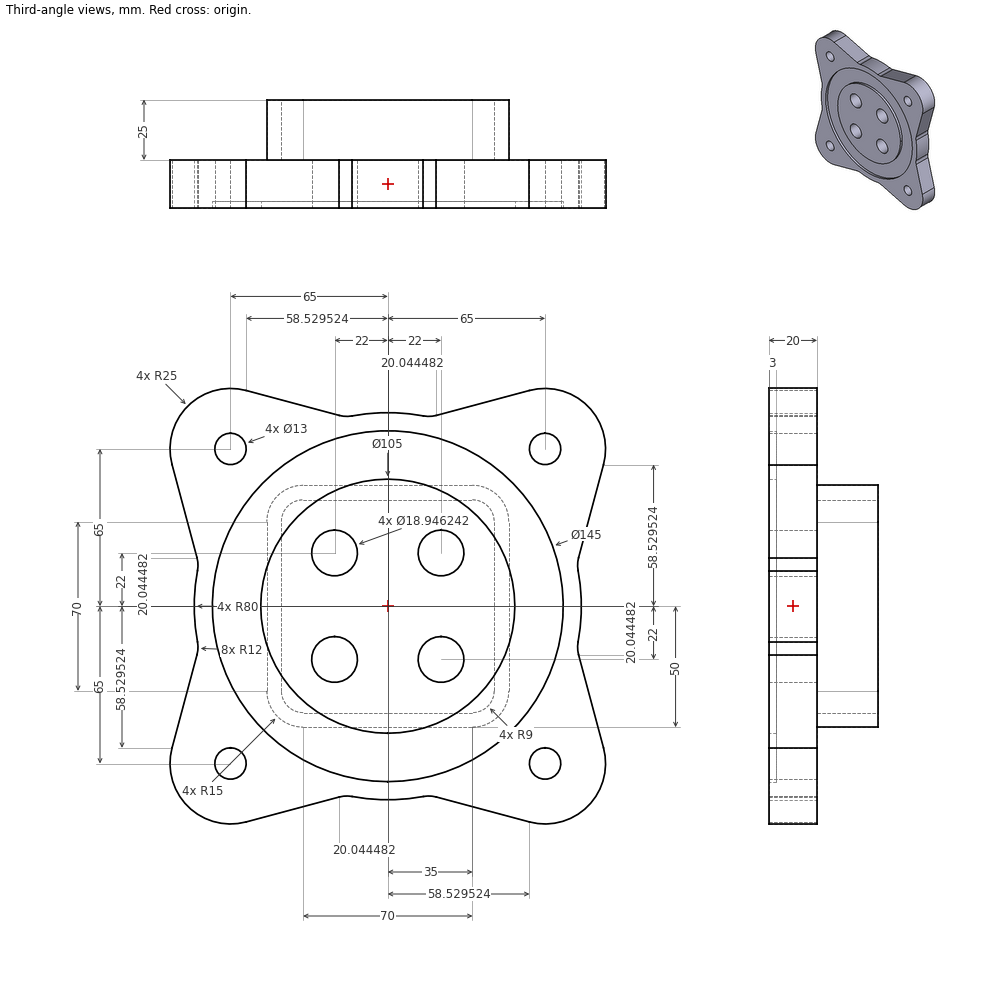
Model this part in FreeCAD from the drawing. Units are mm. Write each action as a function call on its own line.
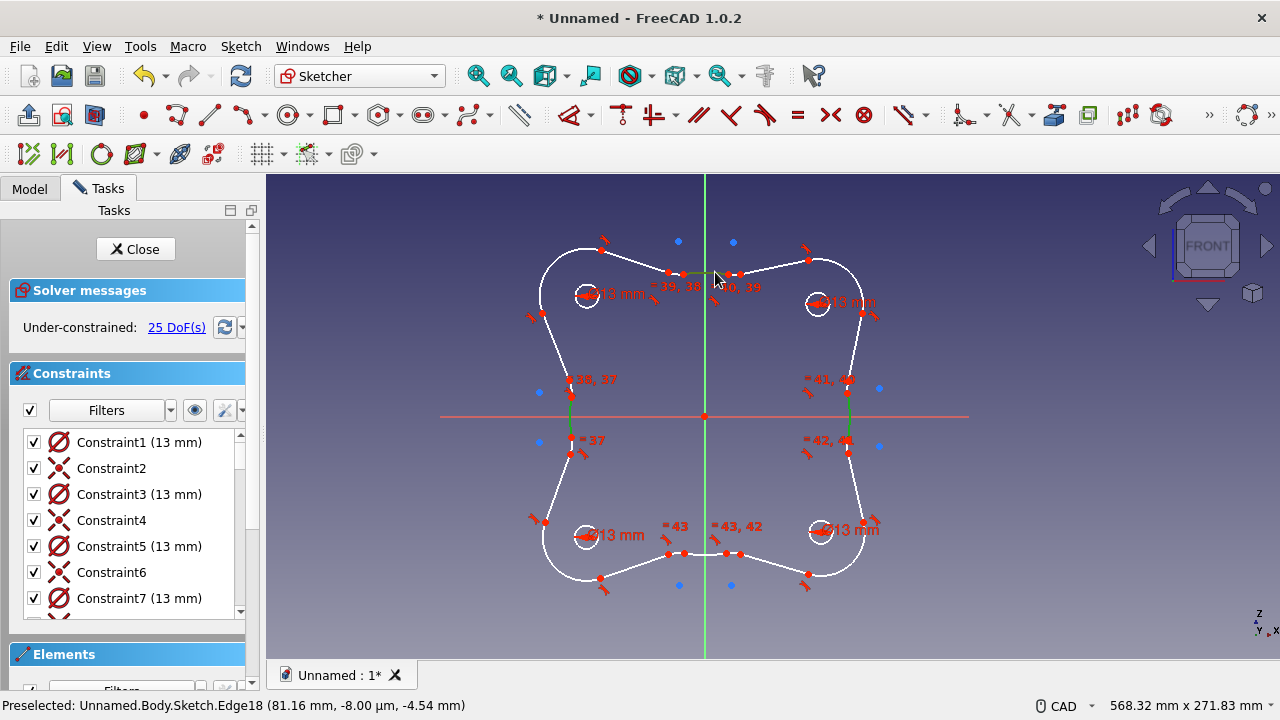
scroll(697, 555, up, 3)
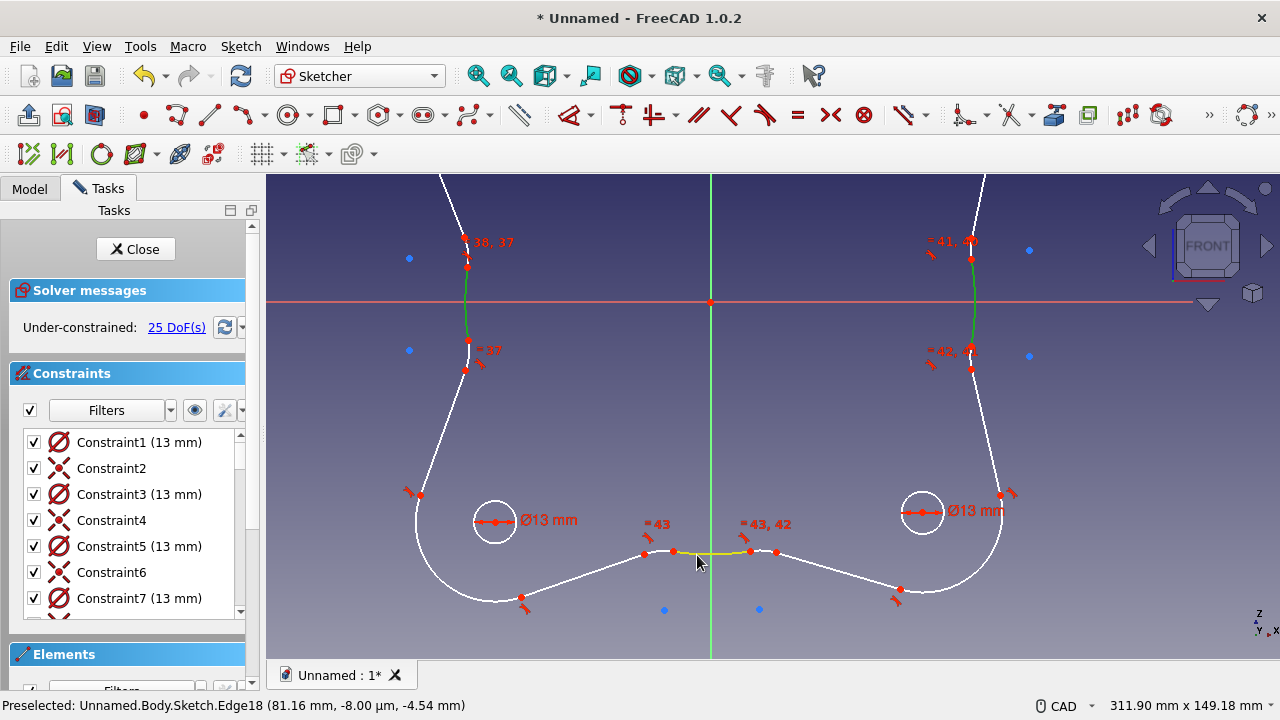
click(696, 554)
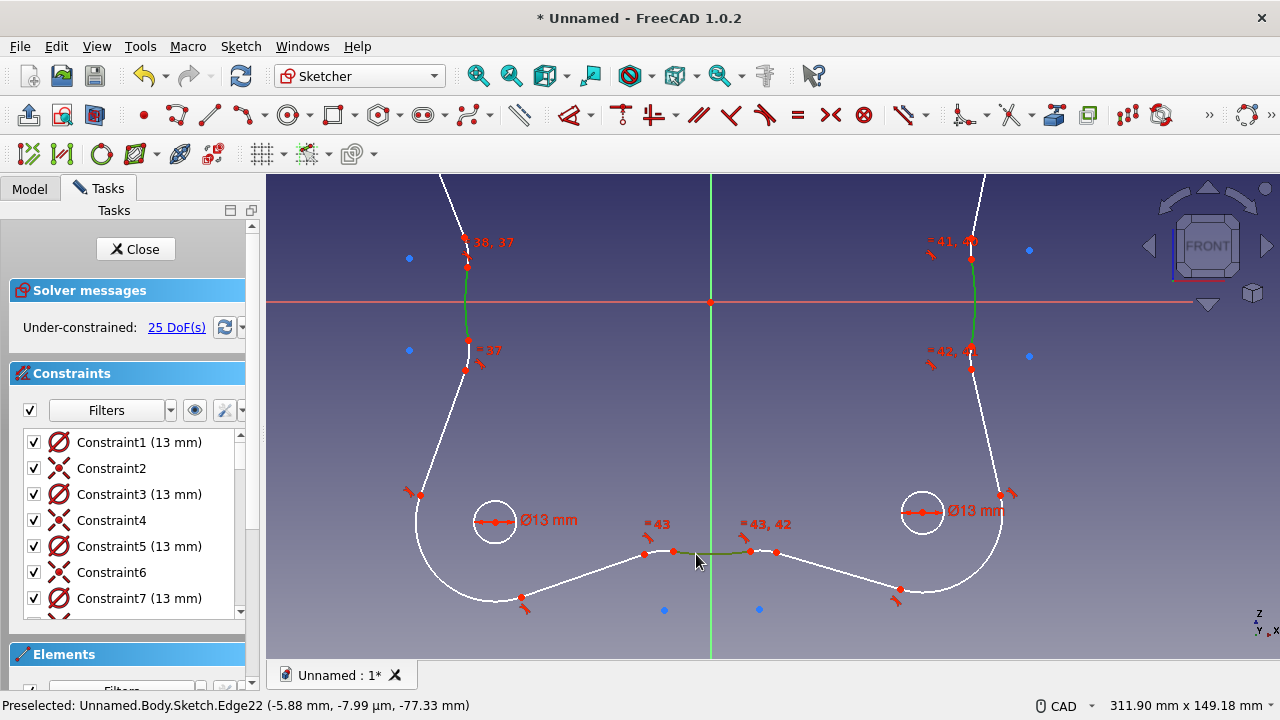
click(798, 116)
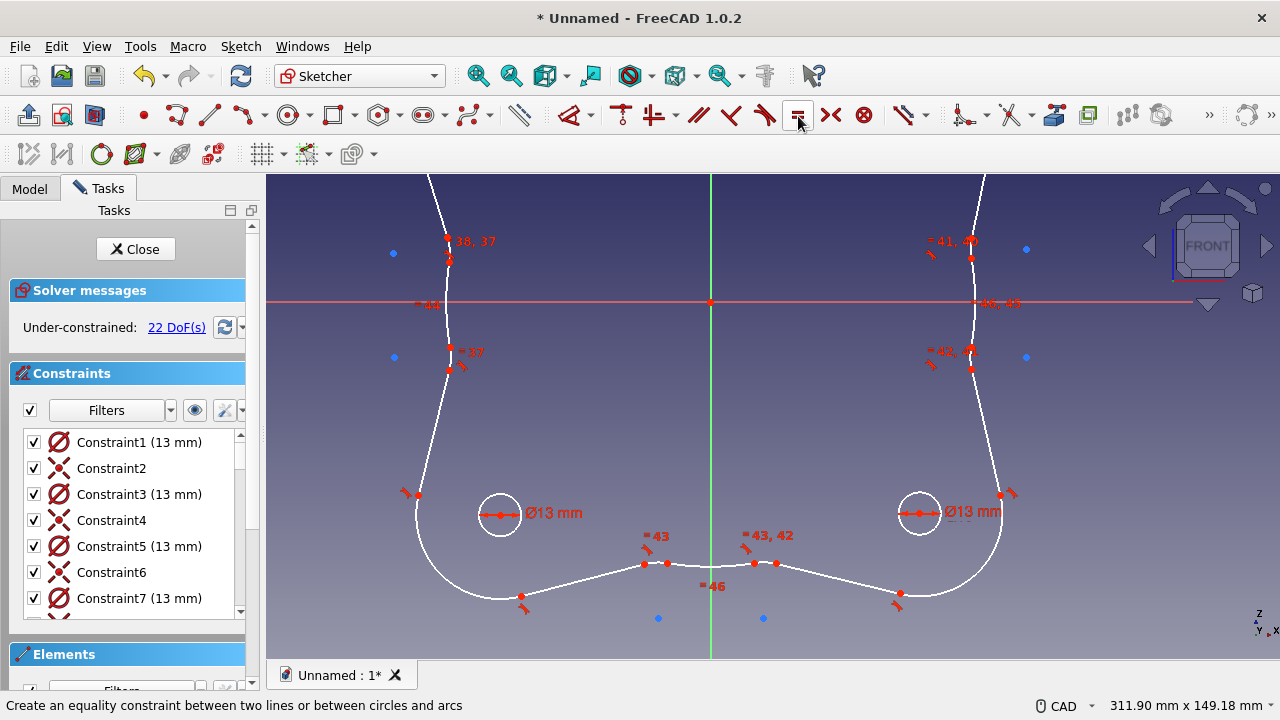
scroll(697, 555, down, 3)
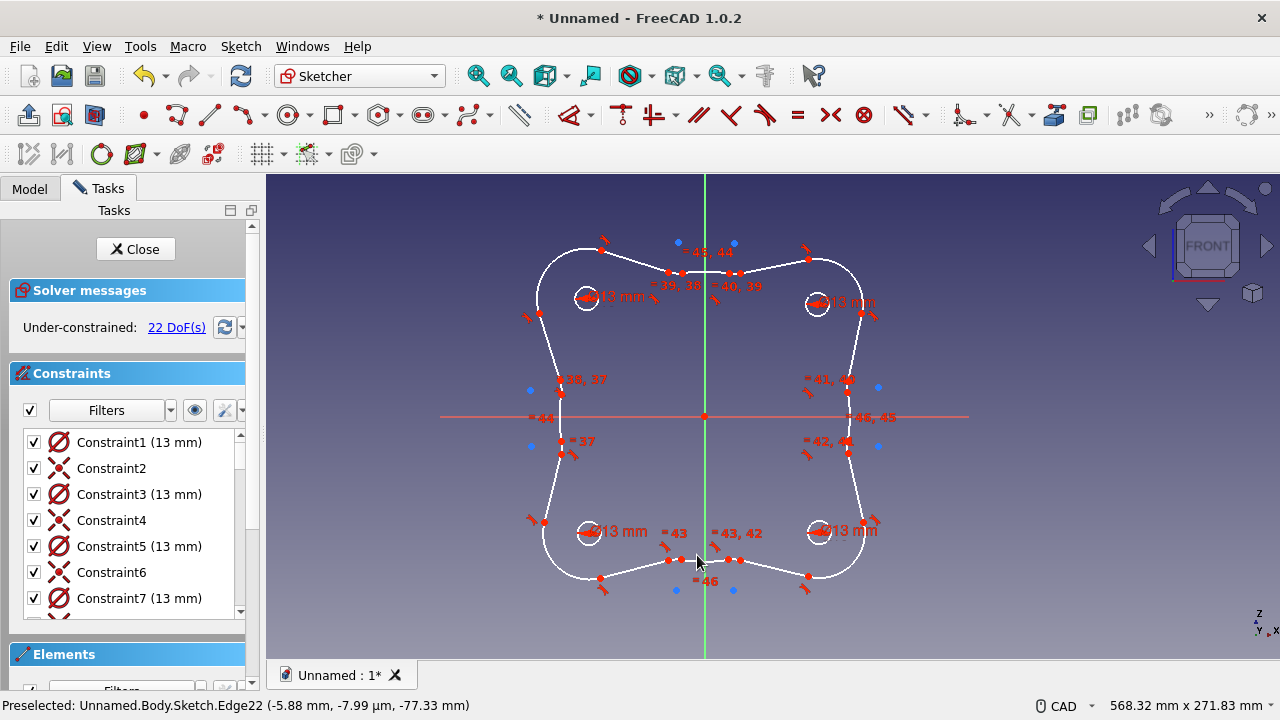
click(570, 252)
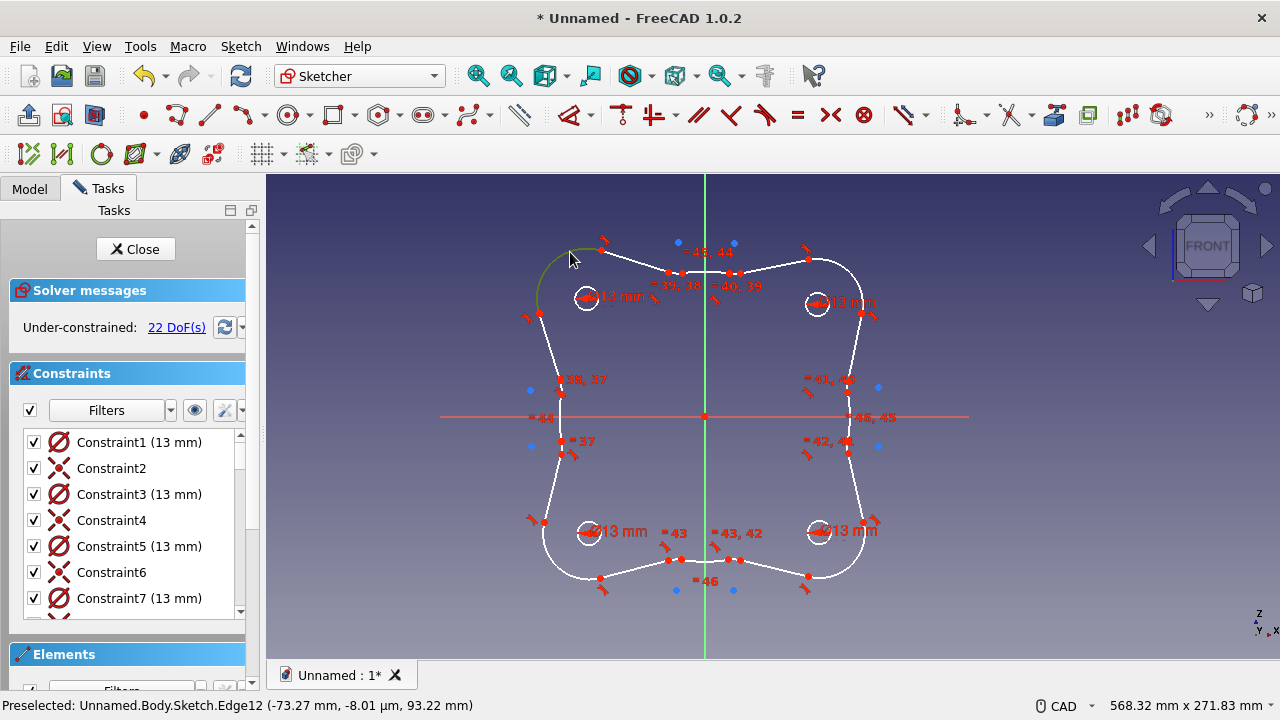
click(859, 287)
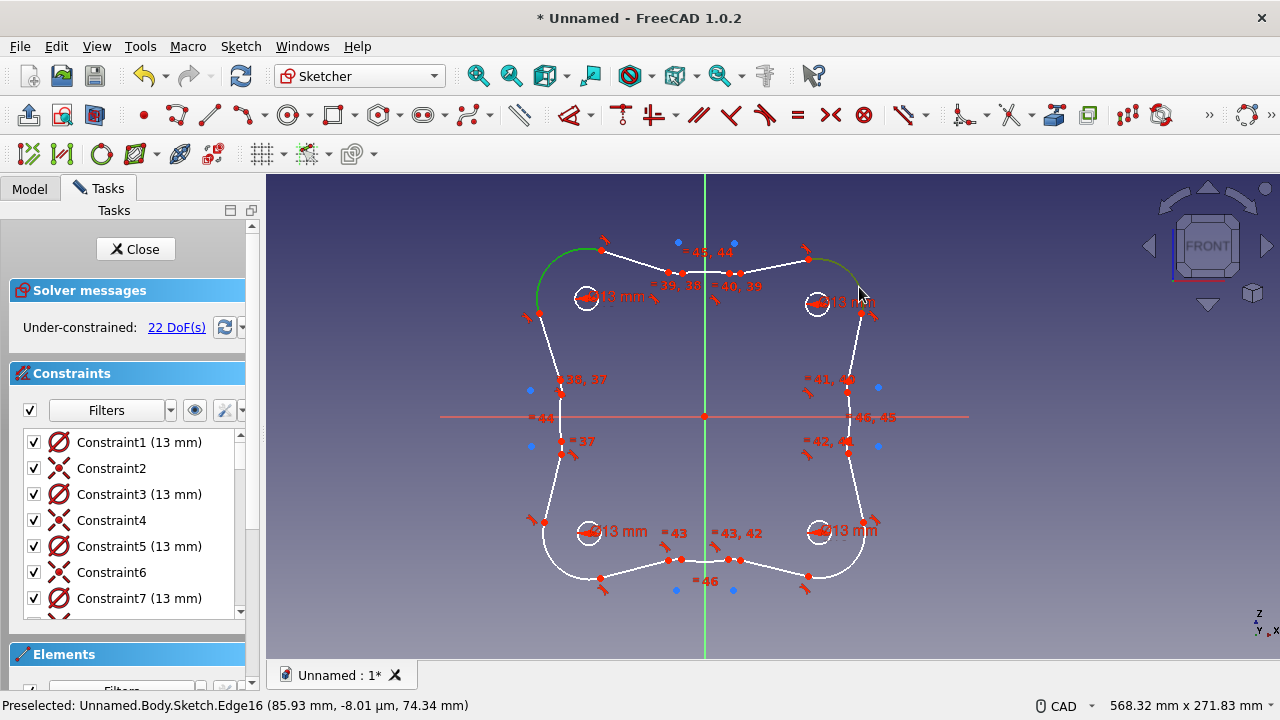
click(836, 575)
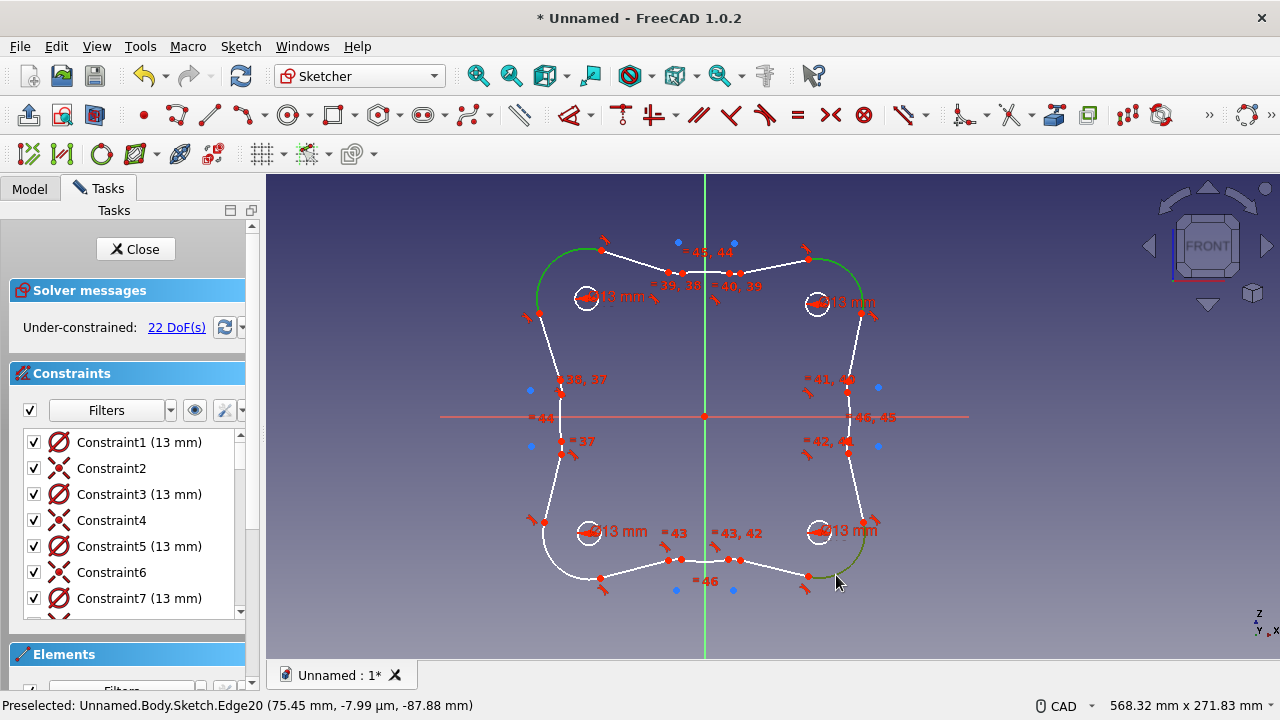
click(546, 551)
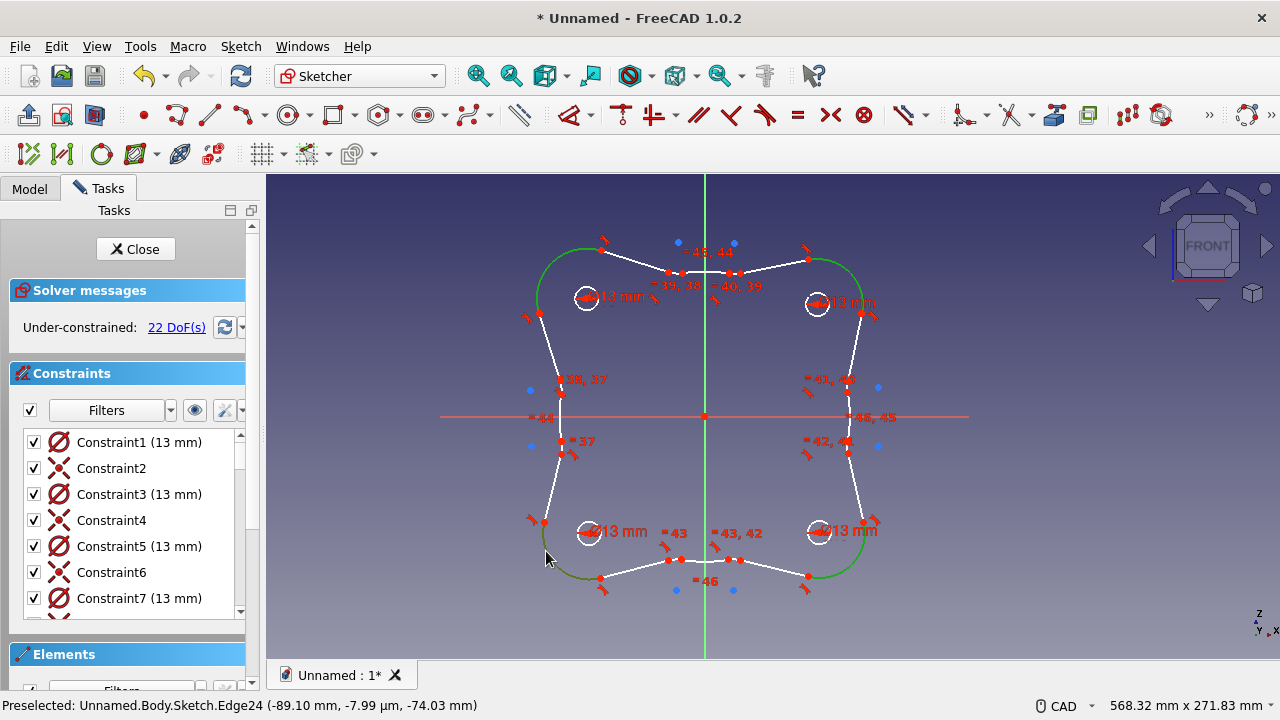
click(798, 116)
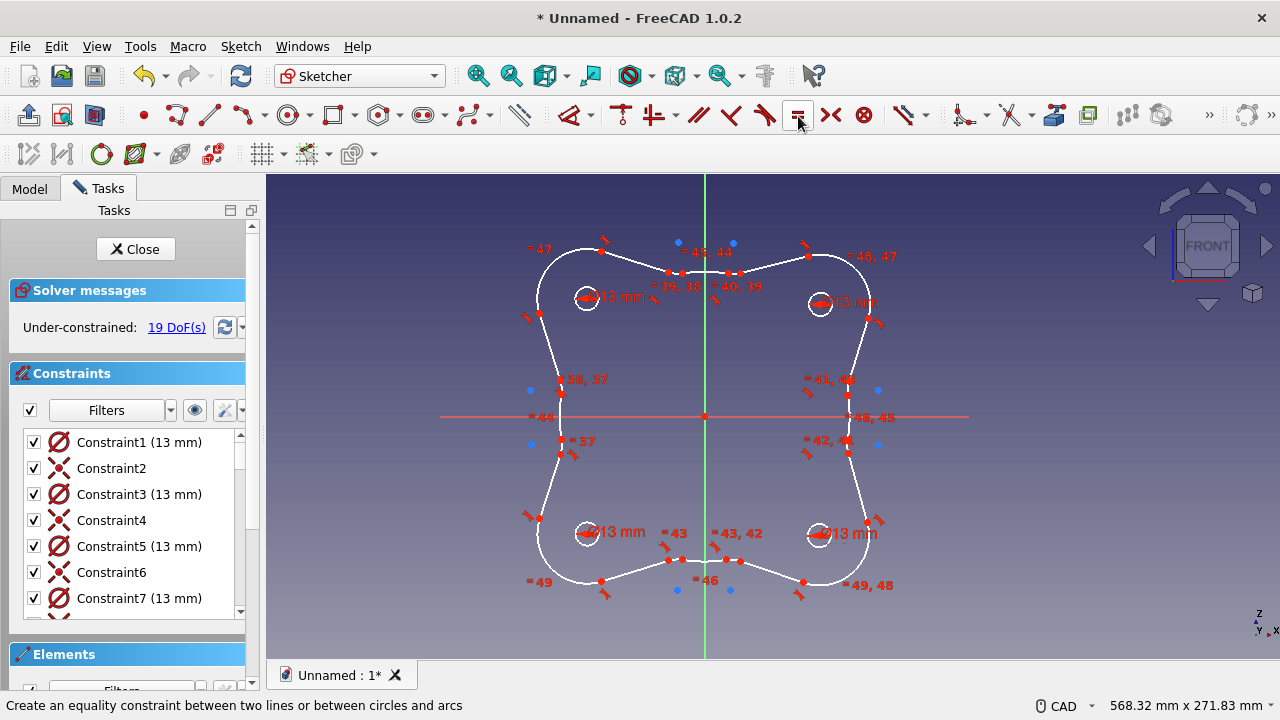
click(568, 116)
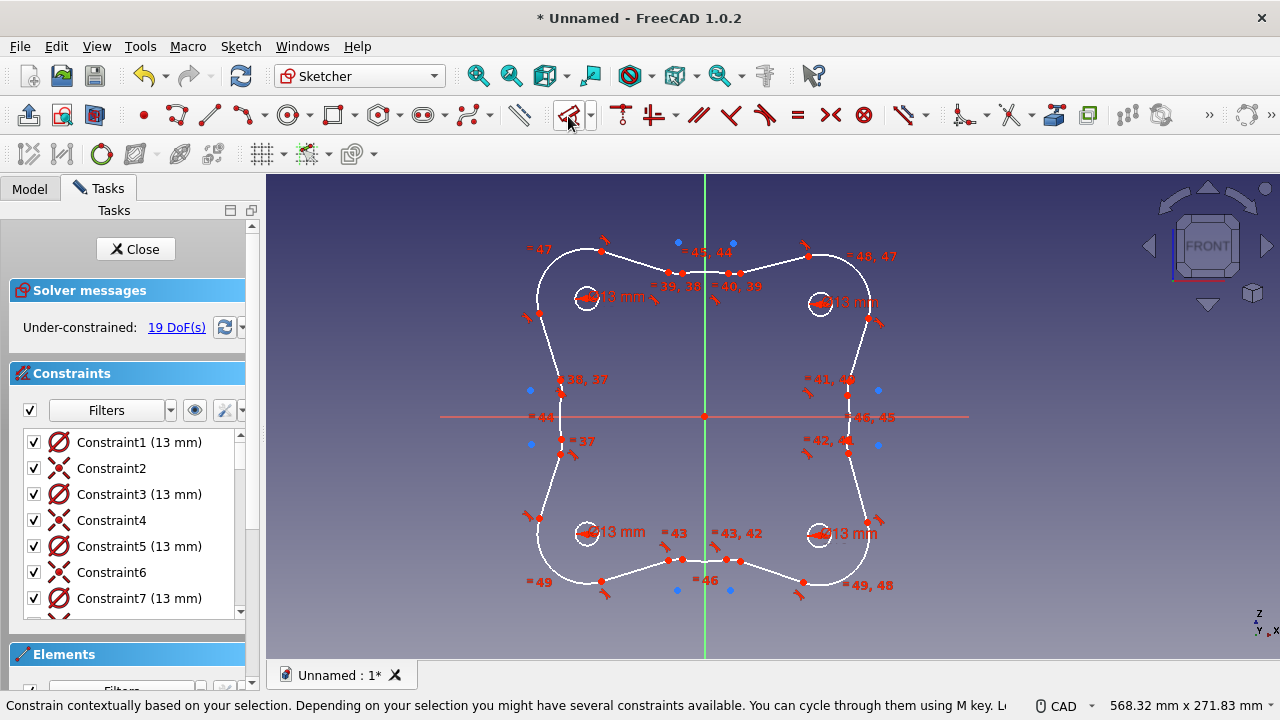
scroll(562, 447, up, 4)